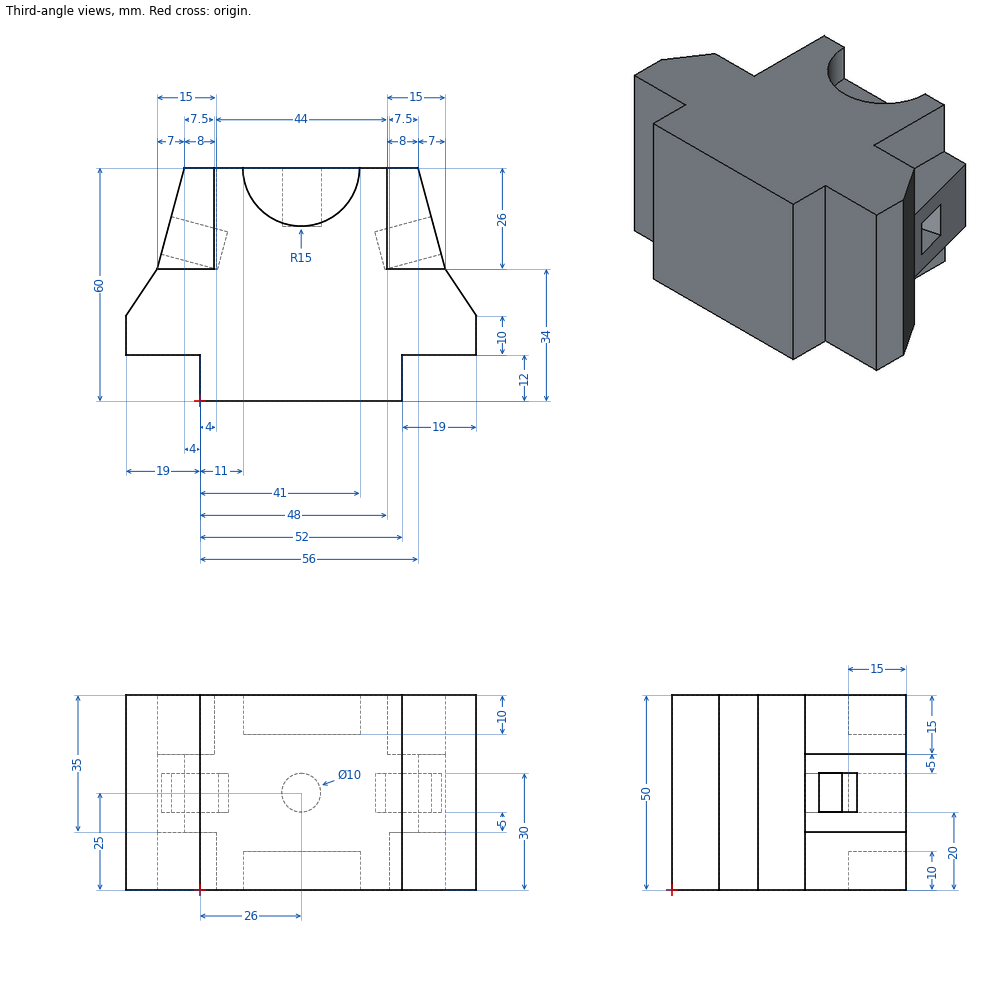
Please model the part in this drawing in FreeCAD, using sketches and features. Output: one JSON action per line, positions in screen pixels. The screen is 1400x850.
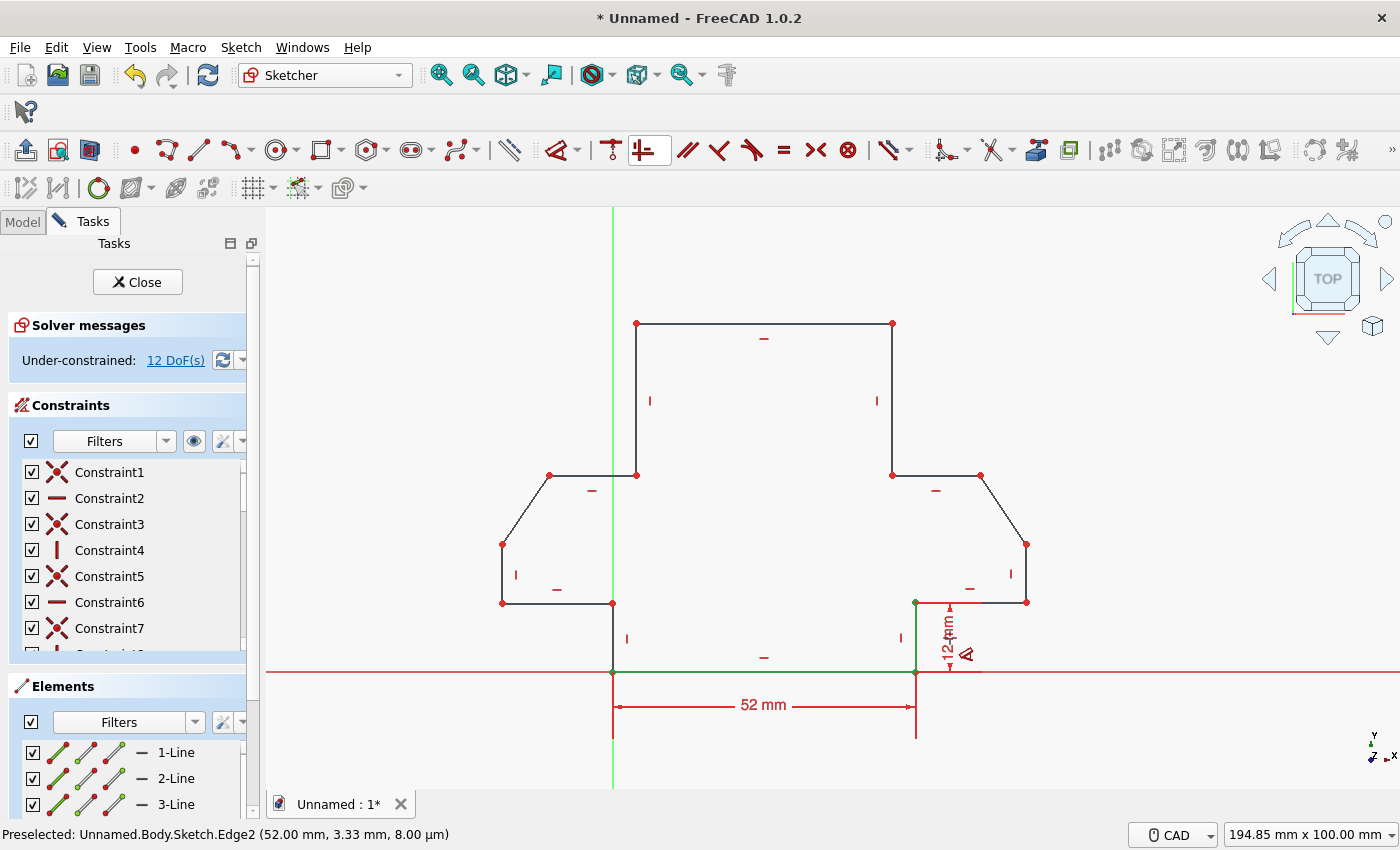
{"action": "left_click", "coordinate": [949, 603]}
{"action": "left_click", "coordinate": [971, 569]}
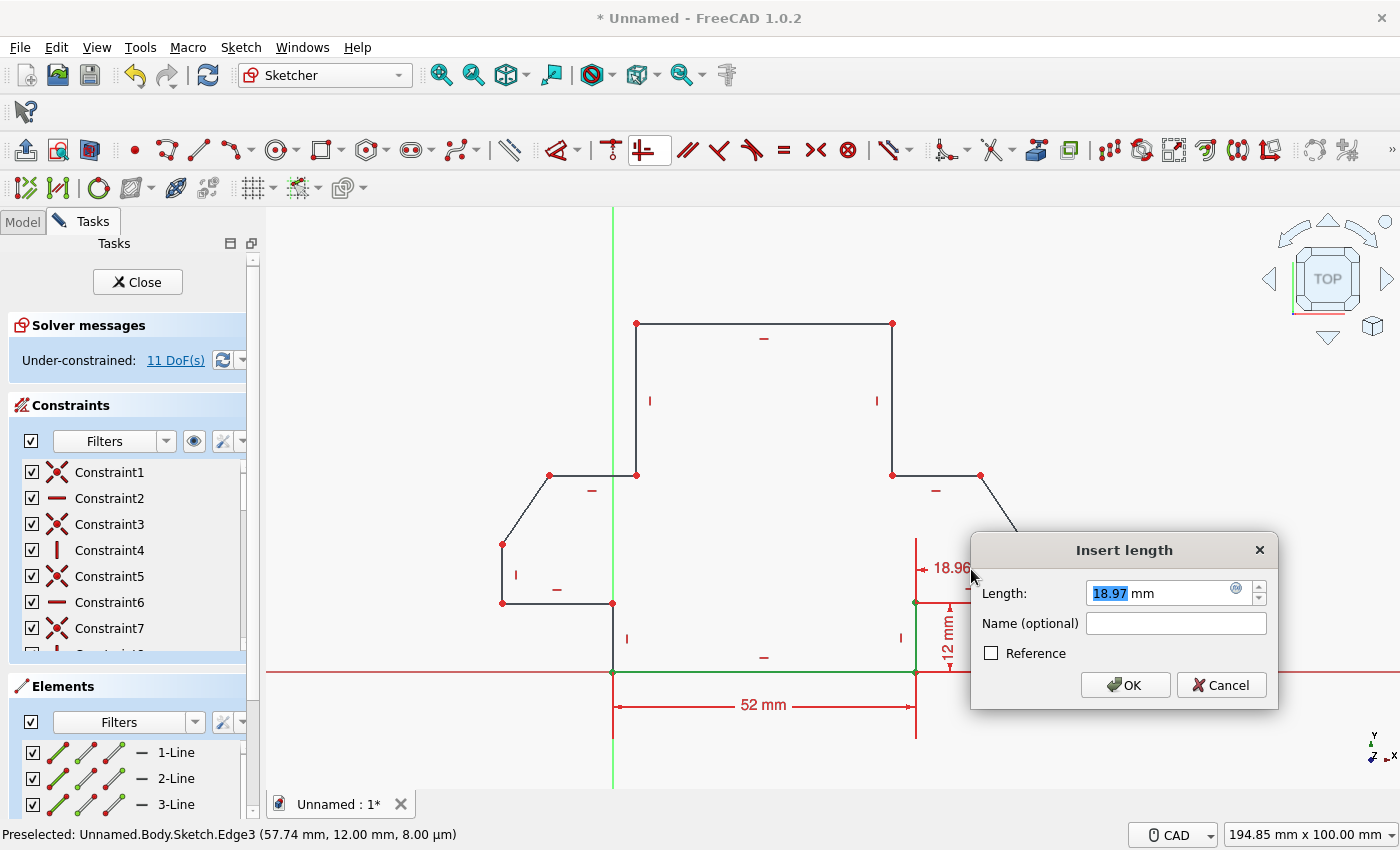
{"action": "type", "text": "19"}
{"action": "key", "text": "Return"}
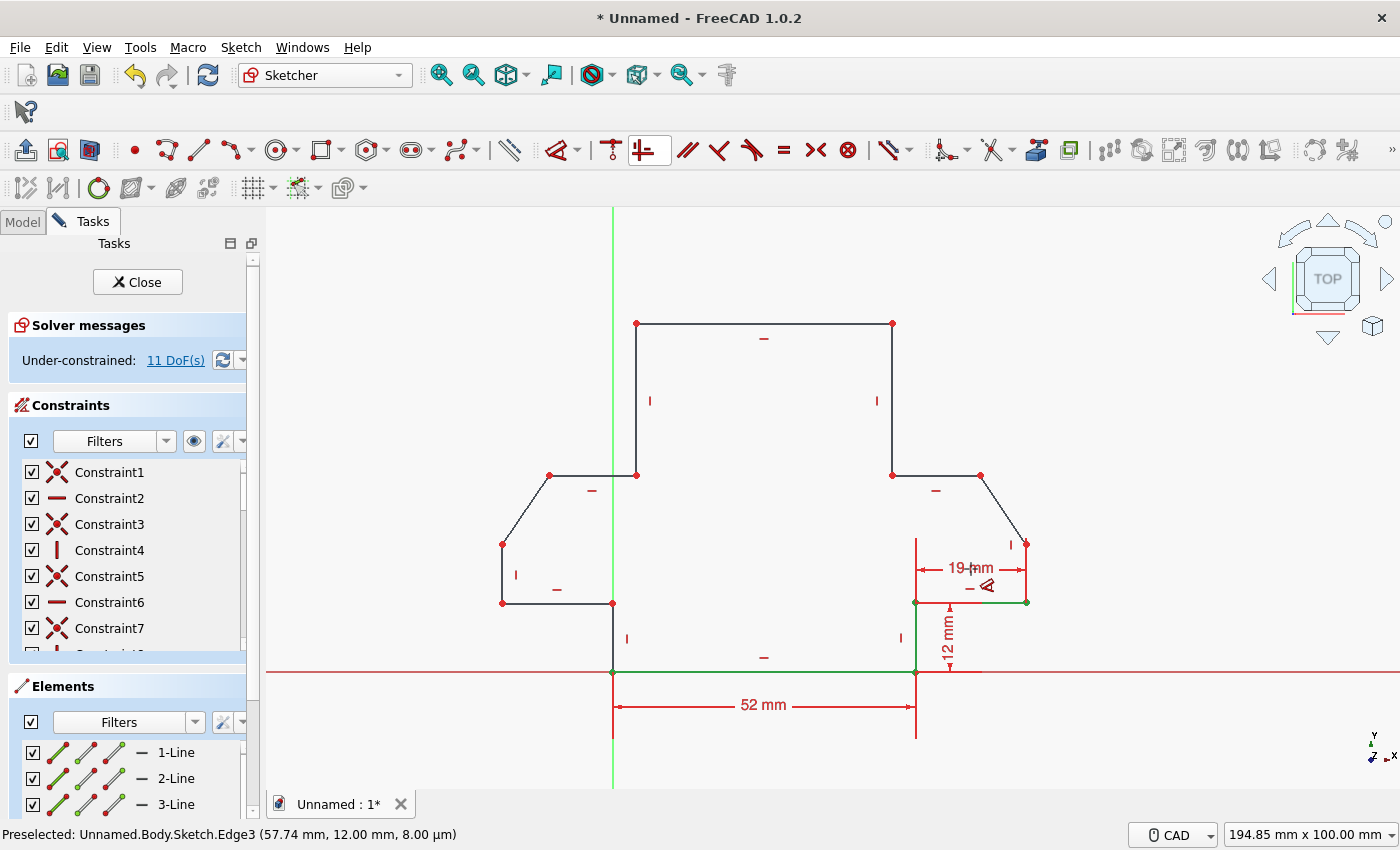
{"action": "left_click", "coordinate": [1026, 585]}
{"action": "left_click", "coordinate": [1060, 574]}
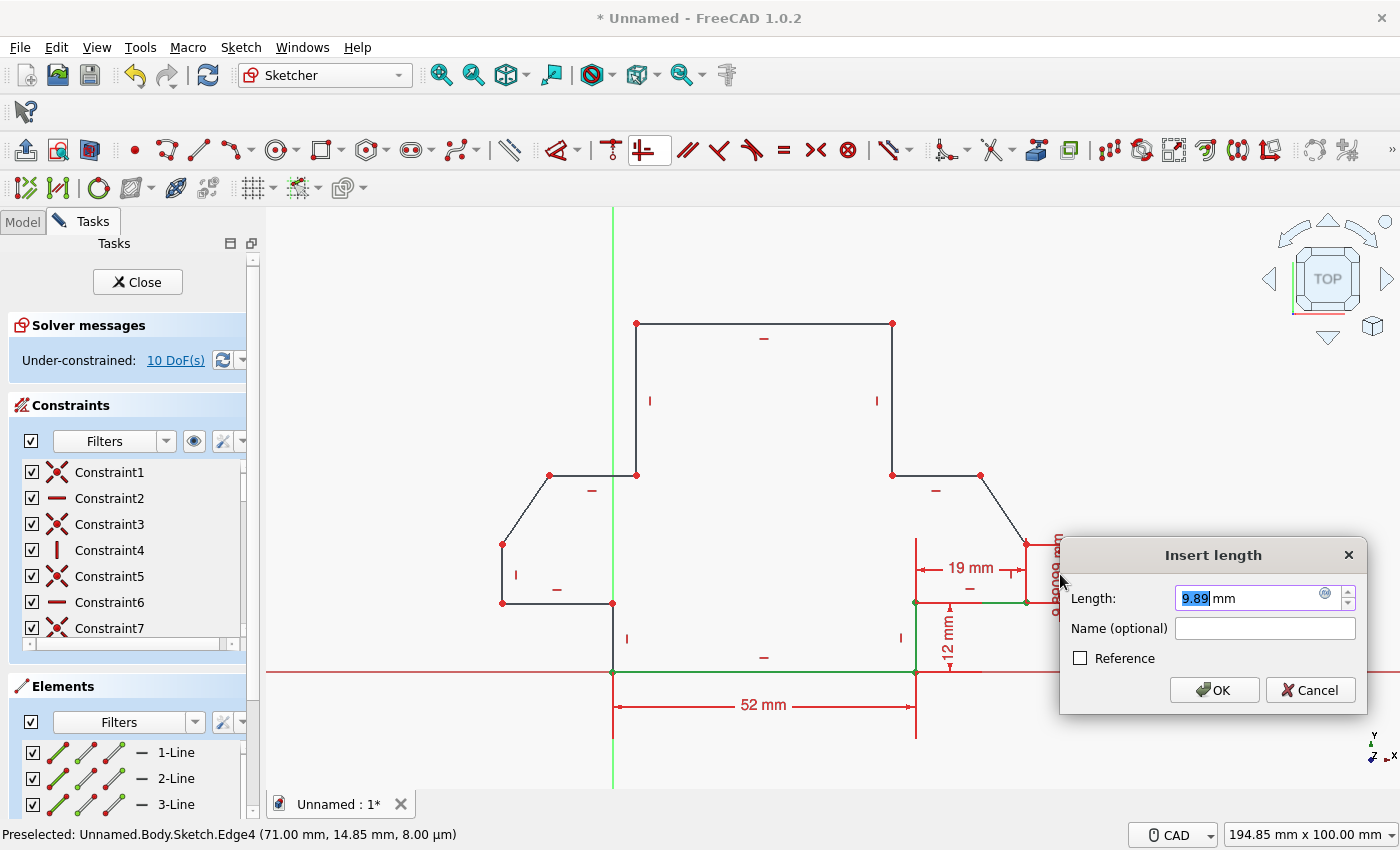
{"action": "type", "text": "10"}
{"action": "key", "text": "Return"}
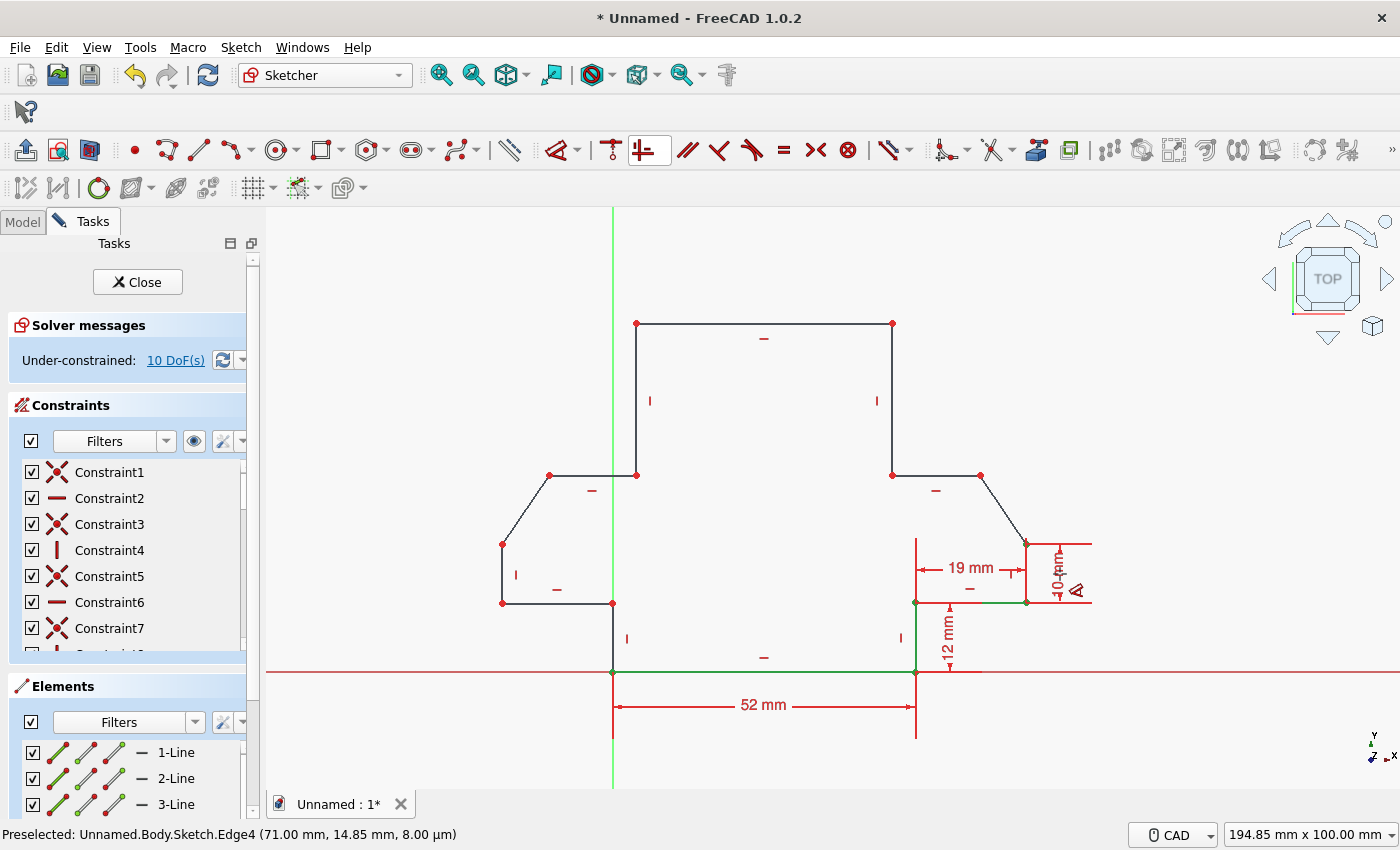
{"action": "left_click", "coordinate": [954, 476]}
{"action": "left_click", "coordinate": [936, 442]}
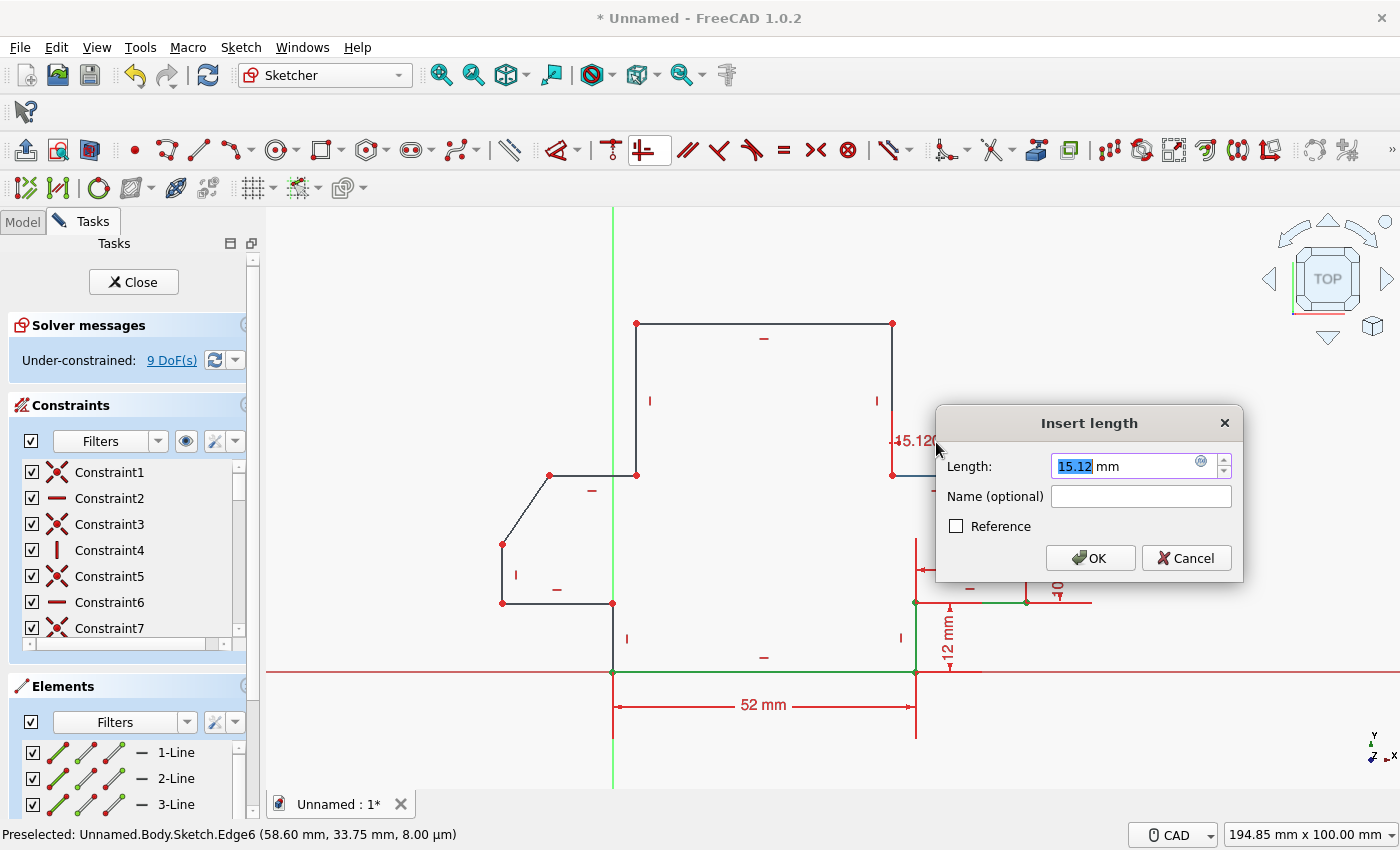
{"action": "type", "text": "15"}
{"action": "key", "text": "Return"}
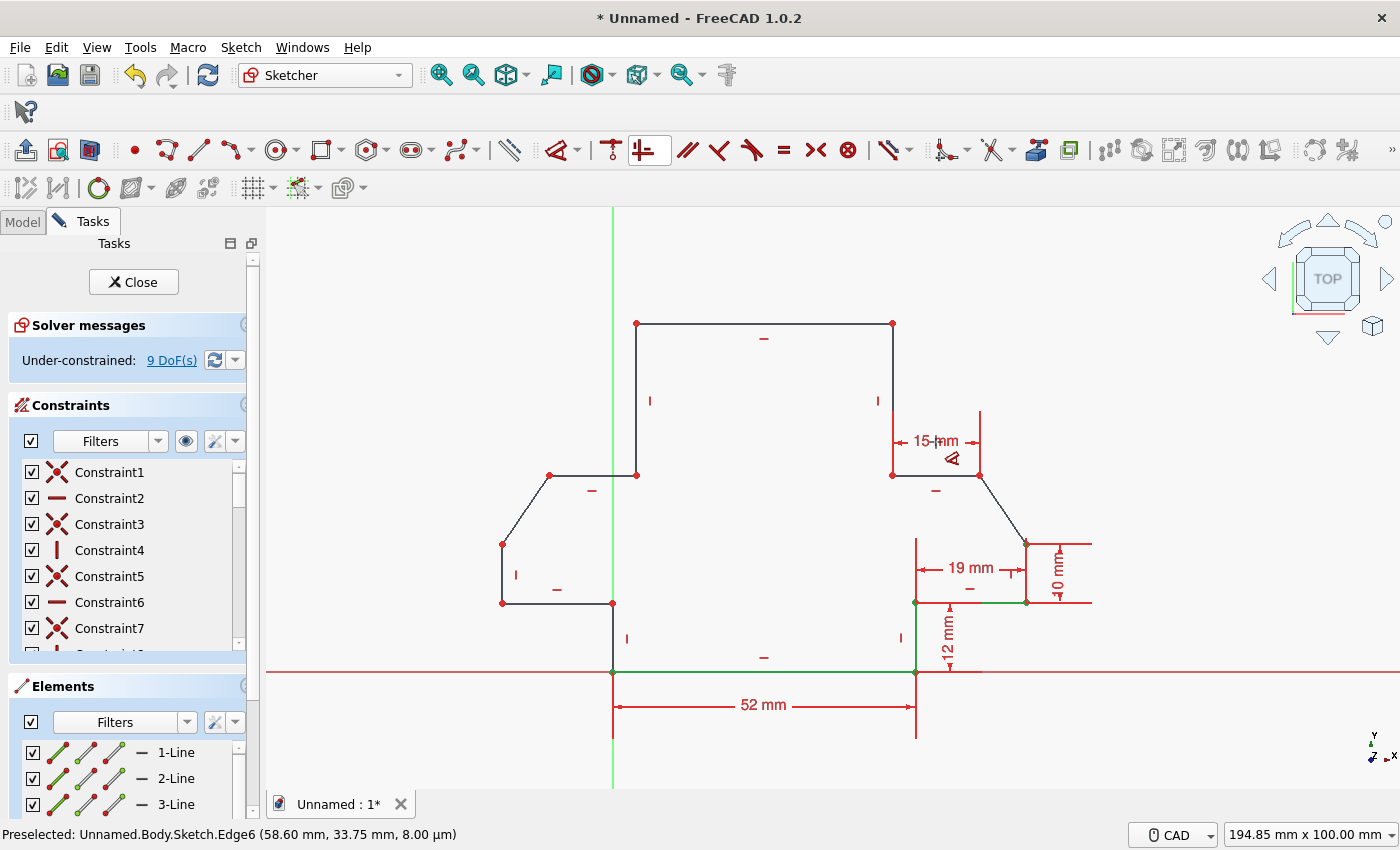
{"action": "left_click", "coordinate": [893, 430]}
{"action": "left_click", "coordinate": [927, 400]}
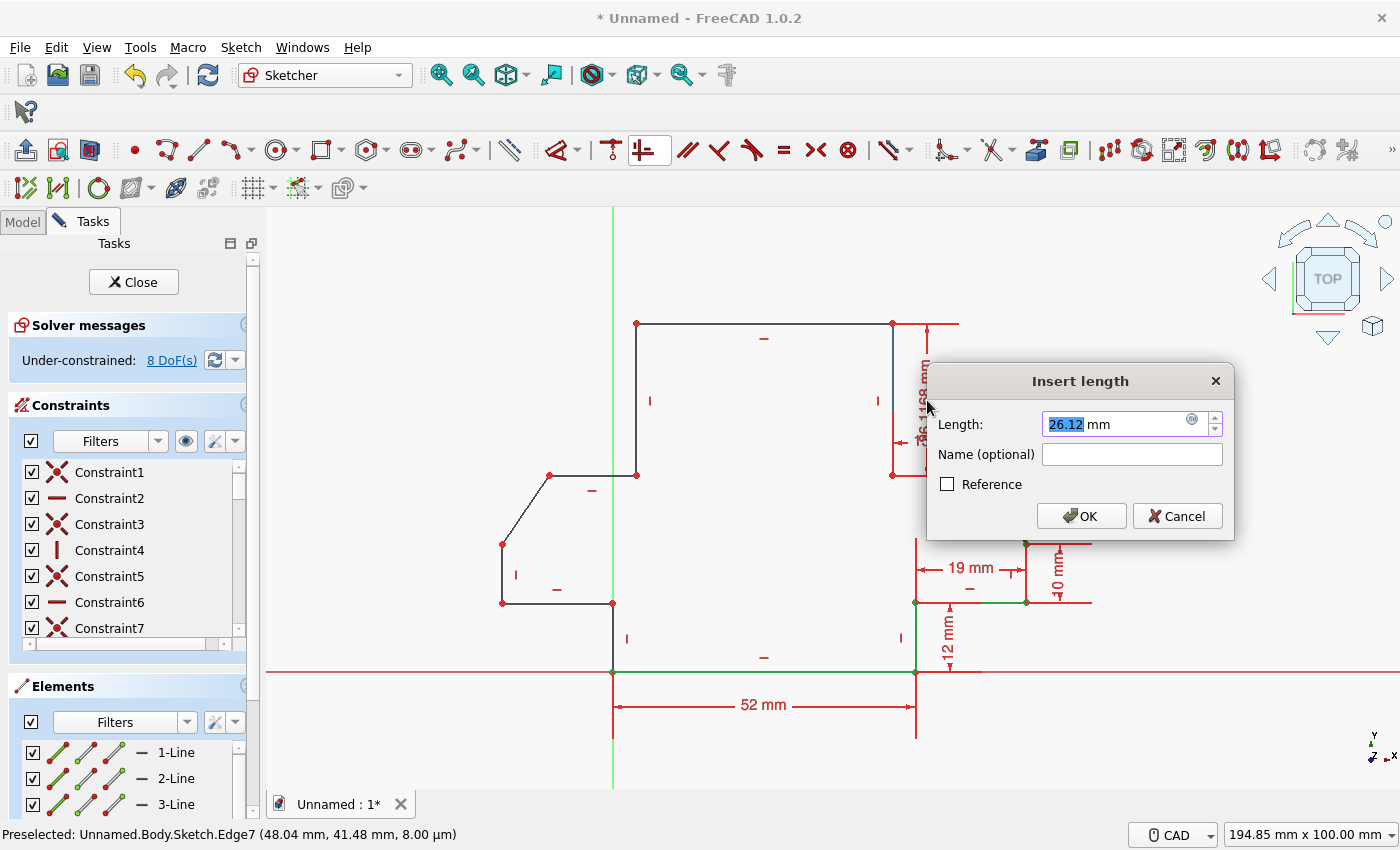
{"action": "type", "text": "26"}
{"action": "key", "text": "Return"}